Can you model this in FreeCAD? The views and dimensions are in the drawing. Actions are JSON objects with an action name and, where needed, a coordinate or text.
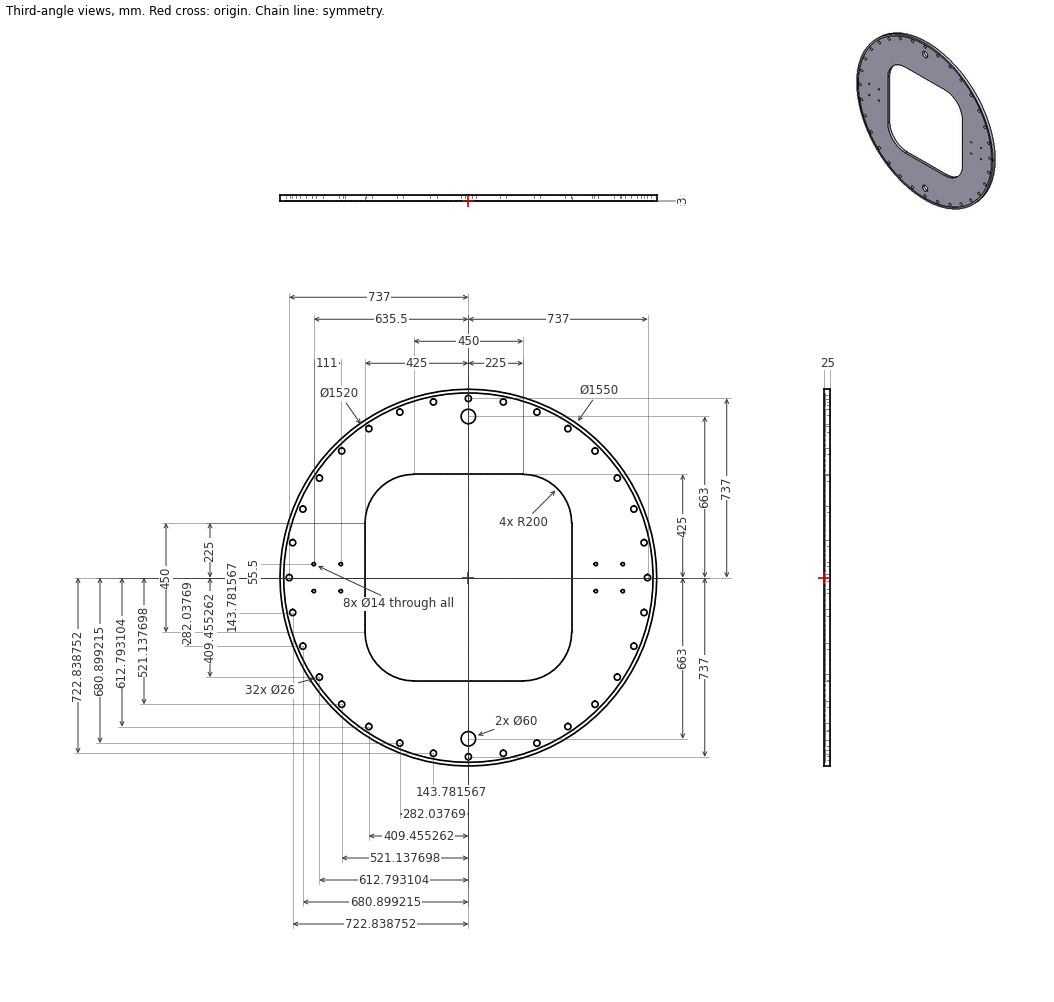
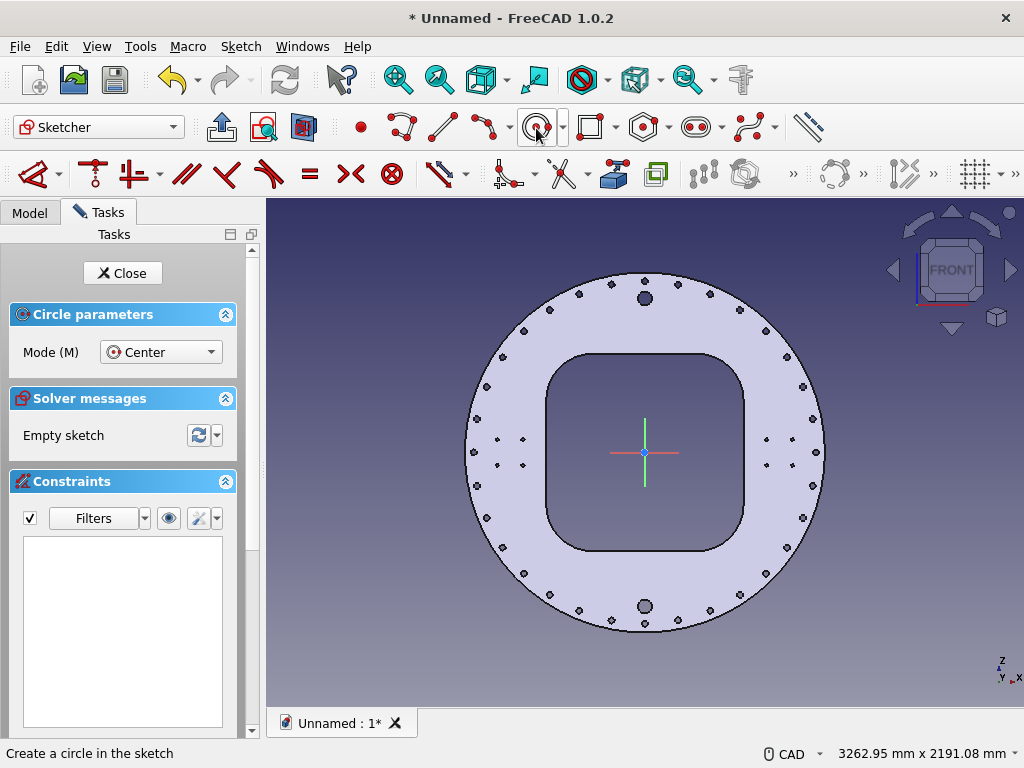
{"action": "left_click", "coordinate": [645, 453]}
{"action": "left_click", "coordinate": [770, 328]}
{"action": "key", "text": "Escape"}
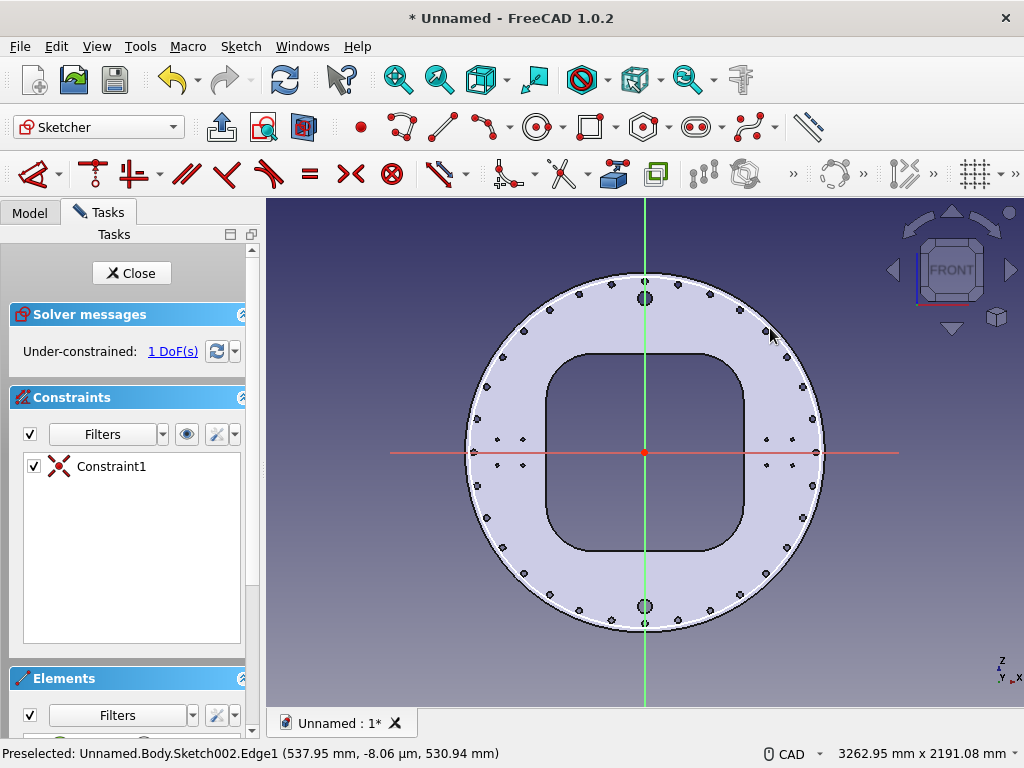
{"action": "left_click", "coordinate": [32, 174]}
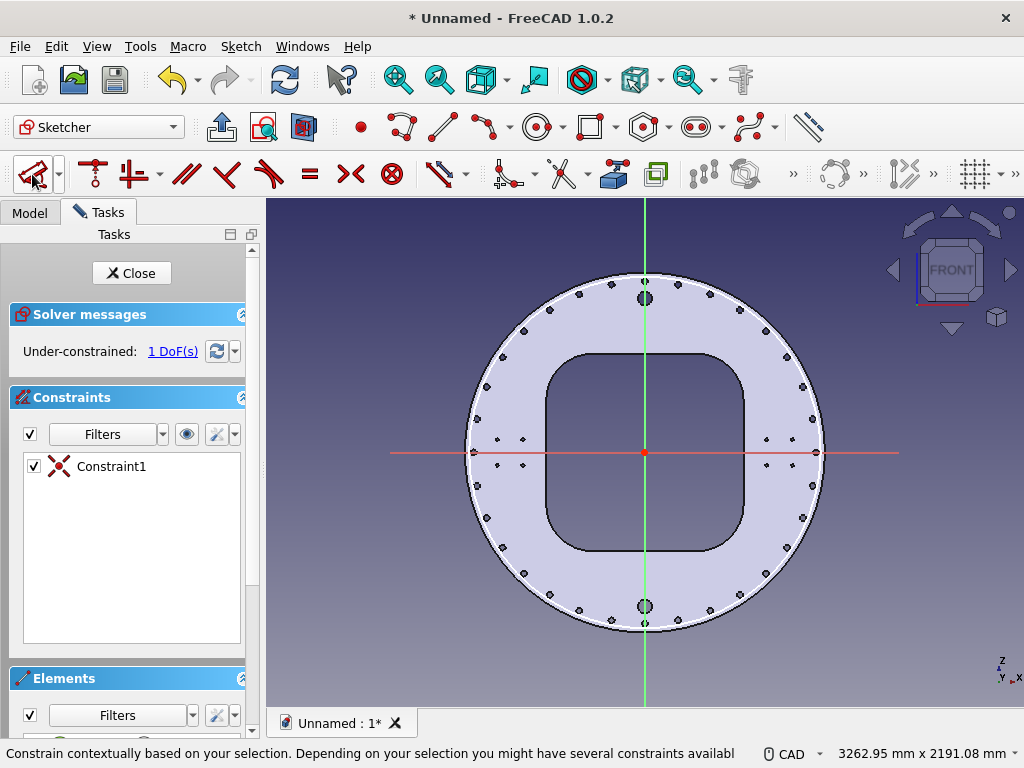
{"action": "left_click", "coordinate": [769, 328]}
{"action": "left_click", "coordinate": [792, 305]}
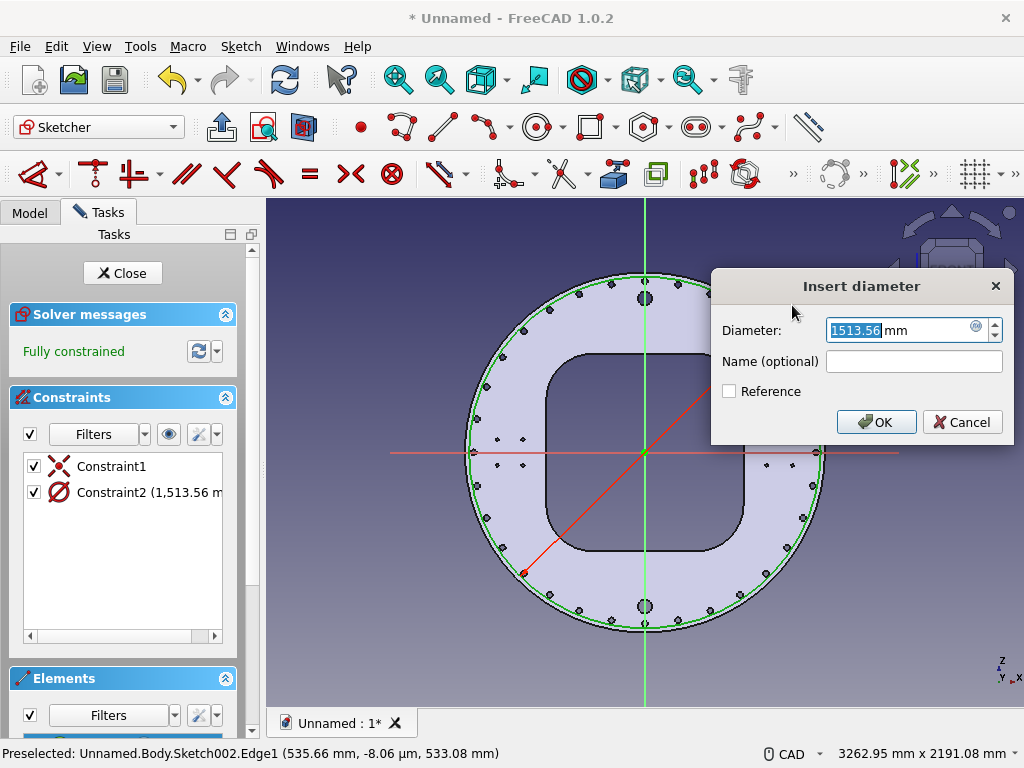
{"action": "type", "text": "1520"}
{"action": "key", "text": "Return"}
{"action": "key", "text": "Escape"}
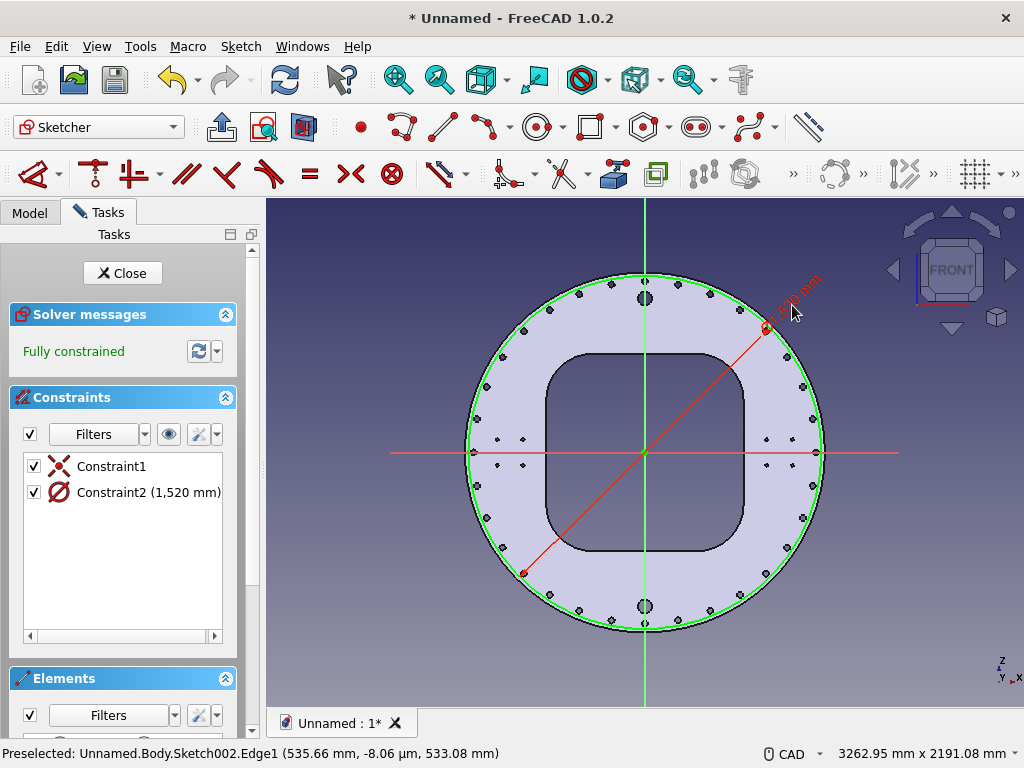
{"action": "left_click", "coordinate": [123, 273]}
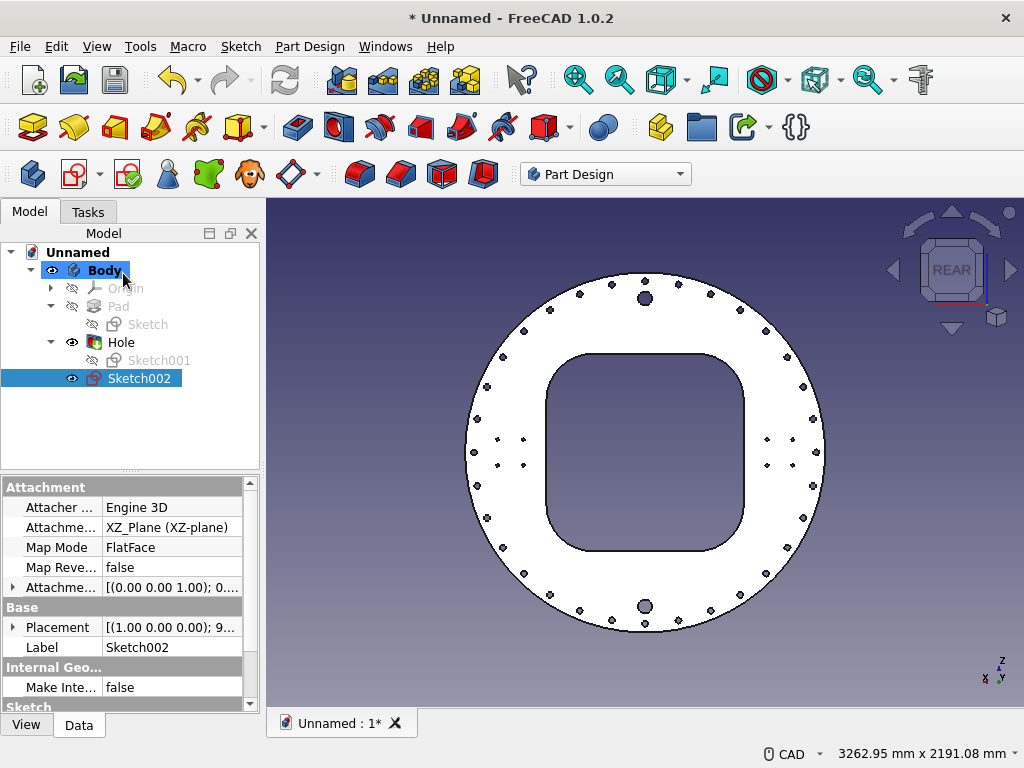
{"action": "left_click", "coordinate": [298, 128]}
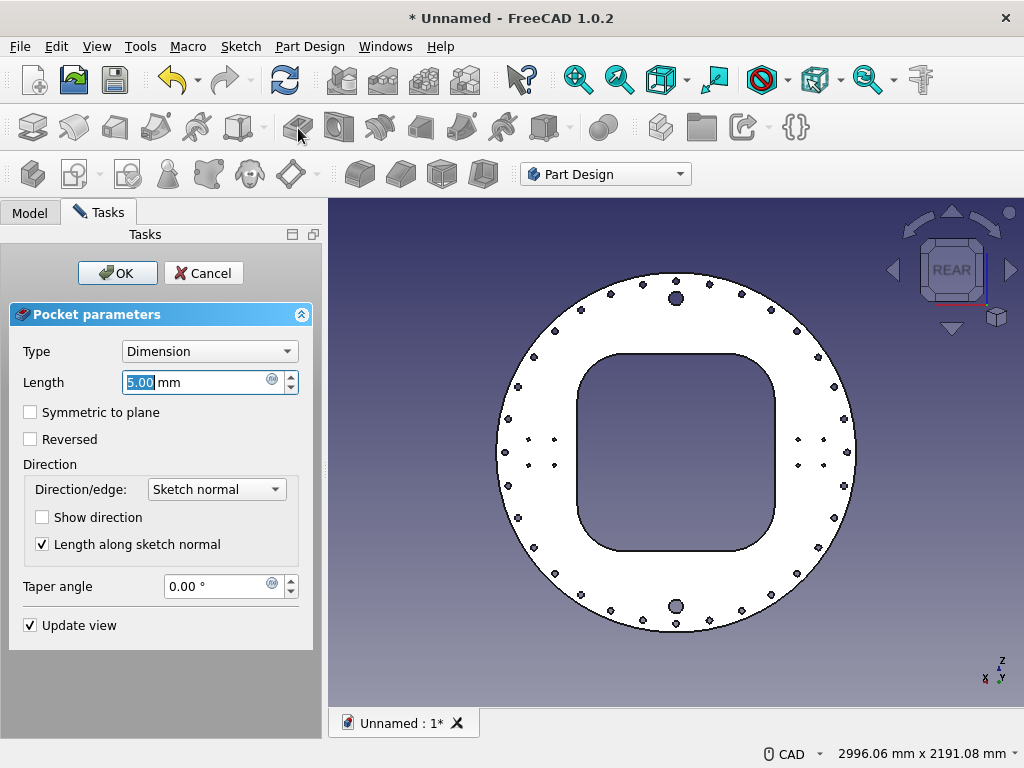
{"action": "type", "text": "3"}
{"action": "key", "text": "Tab"}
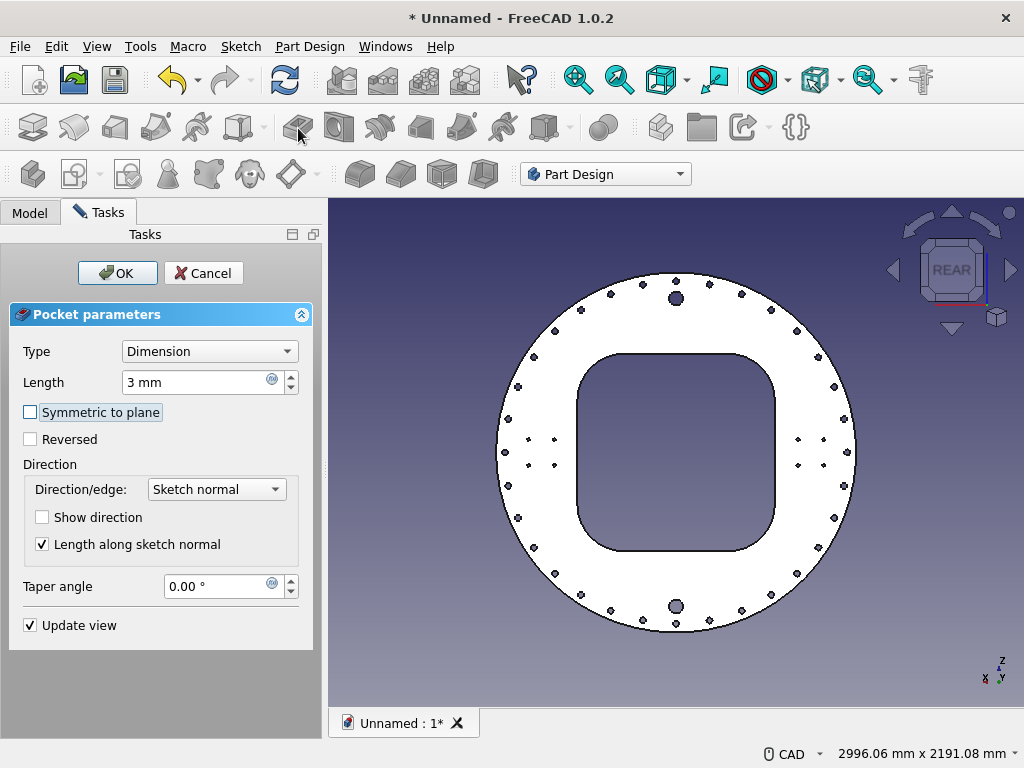
{"action": "left_click", "coordinate": [118, 273]}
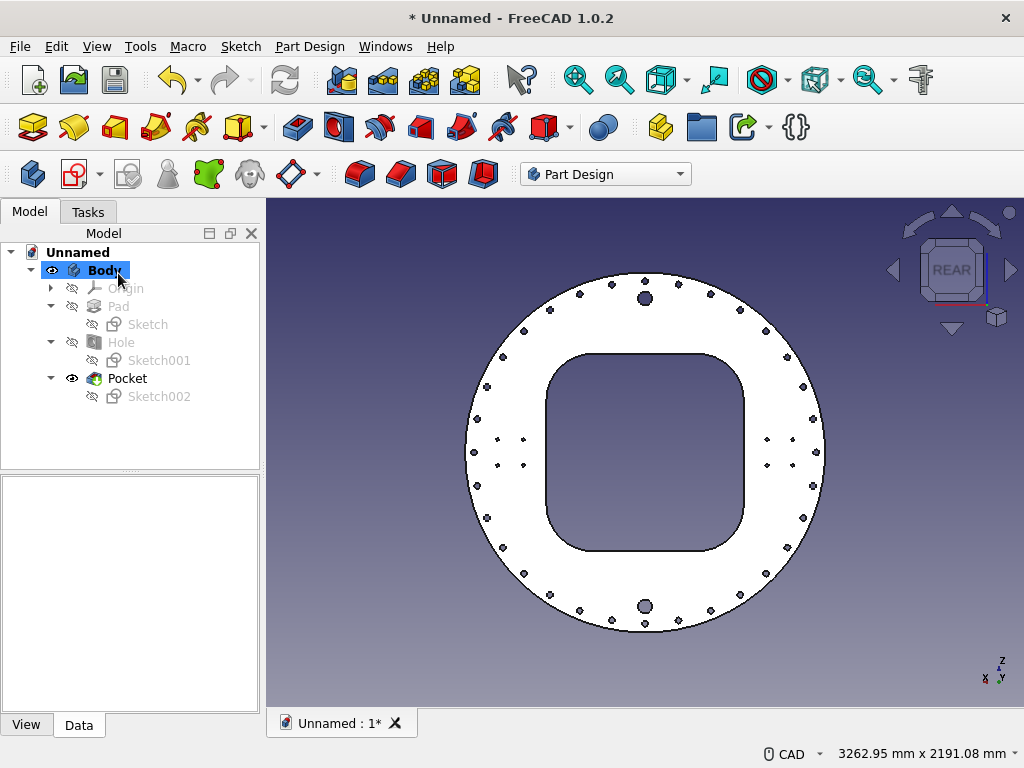
{"action": "key", "text": "0"}